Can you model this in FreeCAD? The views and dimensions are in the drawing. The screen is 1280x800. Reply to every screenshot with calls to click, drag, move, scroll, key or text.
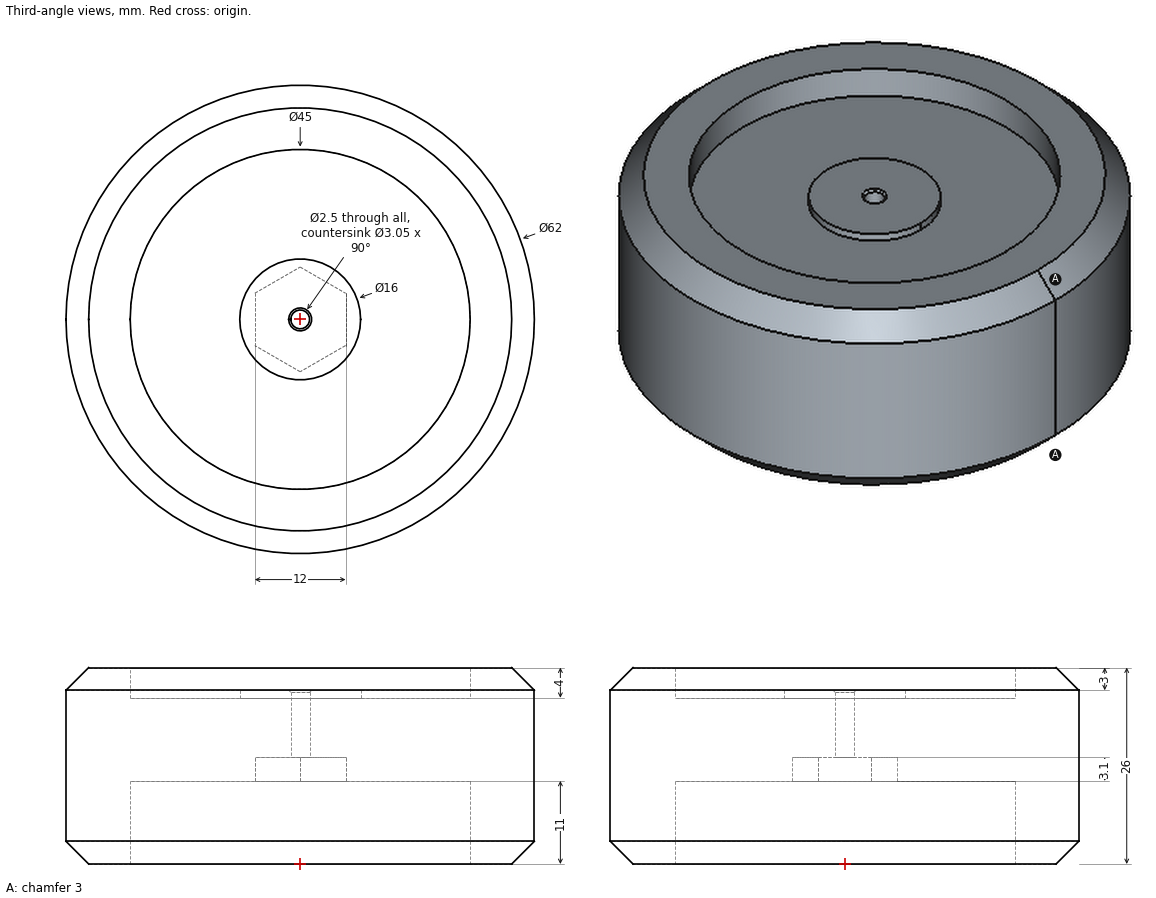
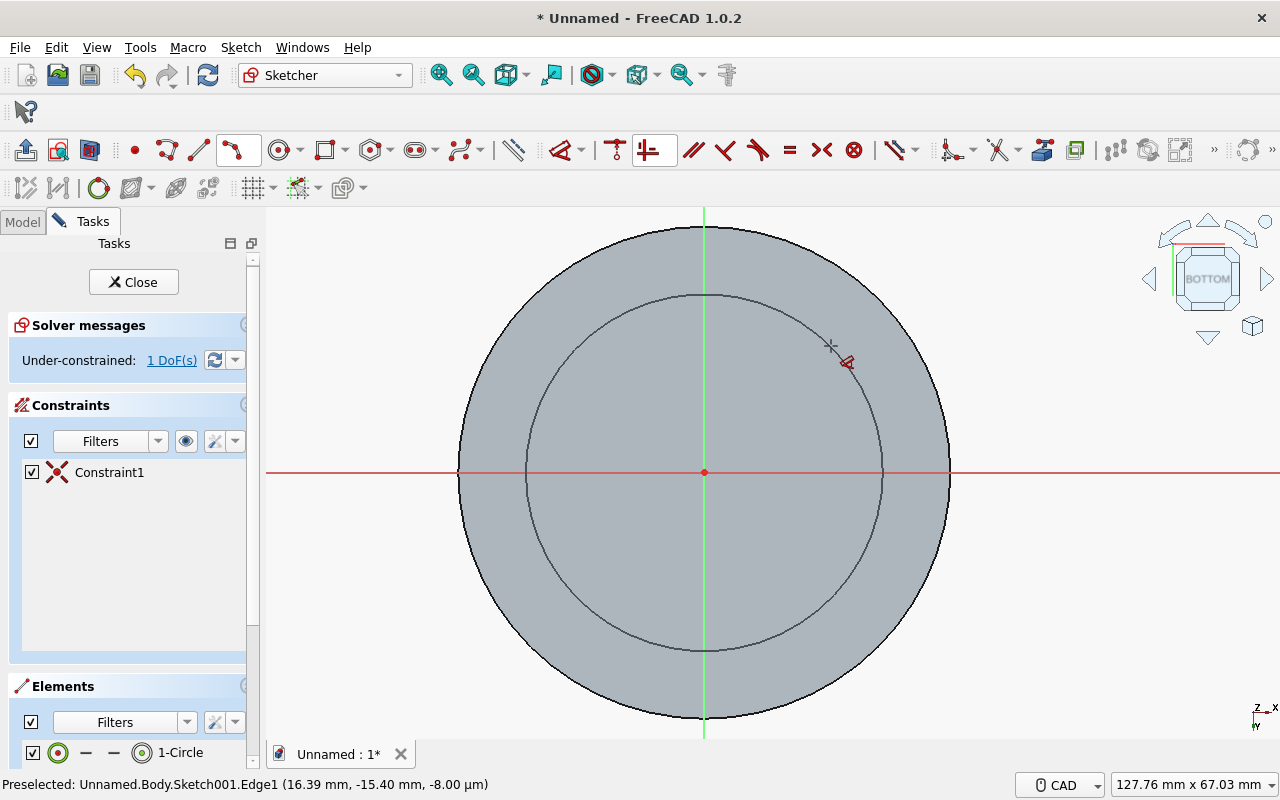
click(830, 346)
click(853, 323)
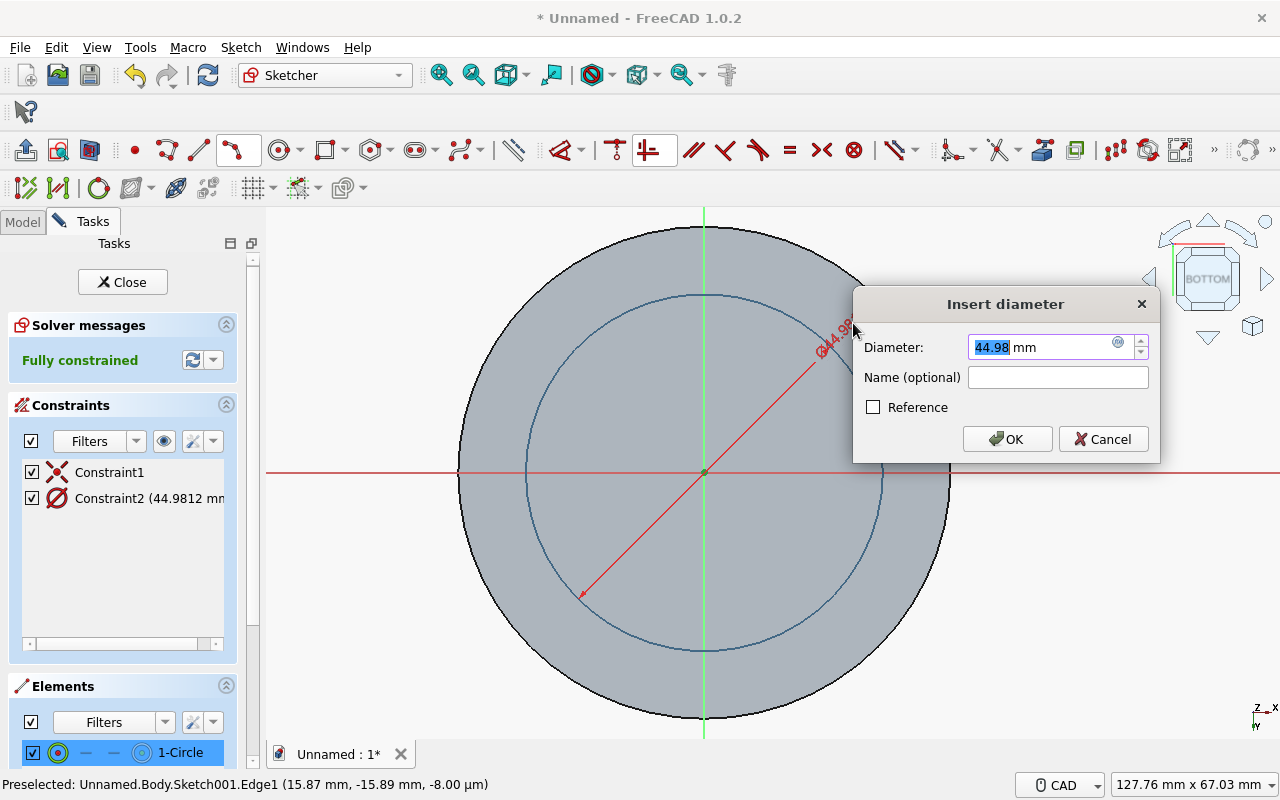
text(45)
key(Return)
key(Escape)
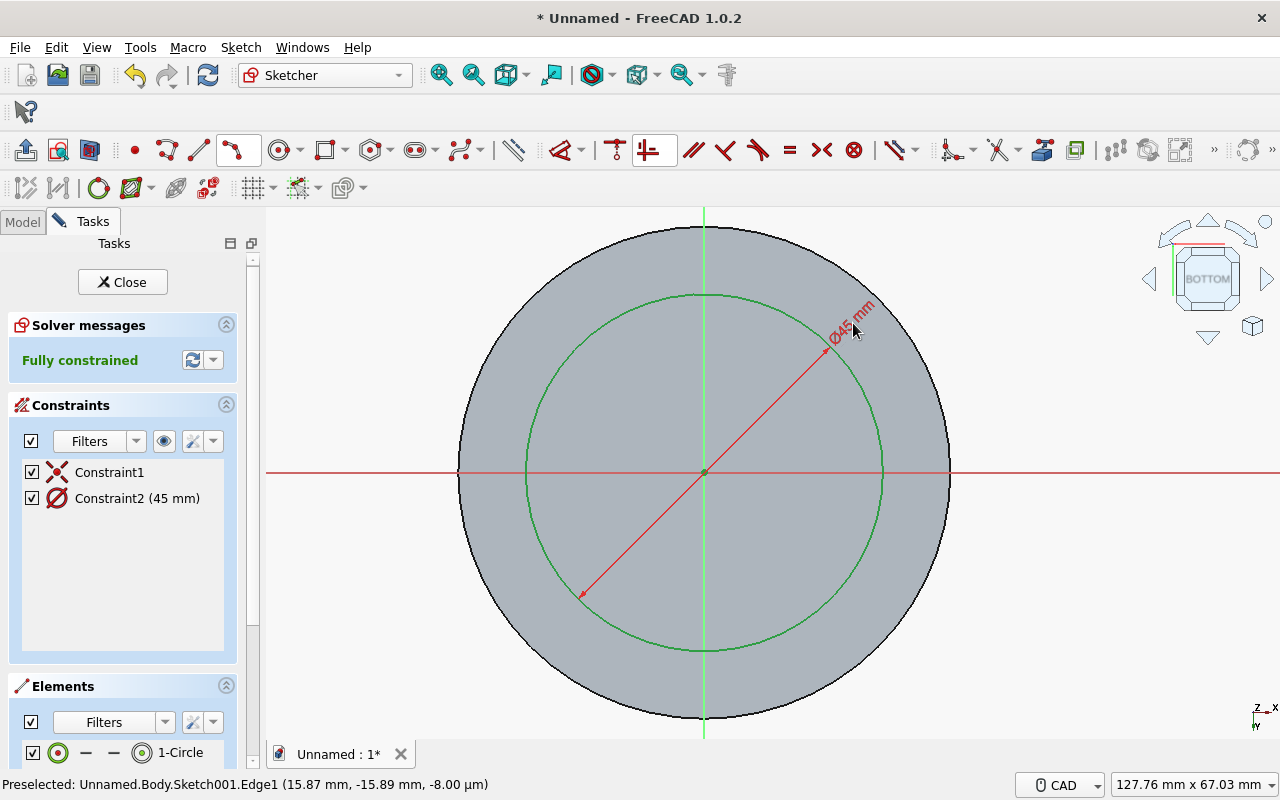
click(123, 282)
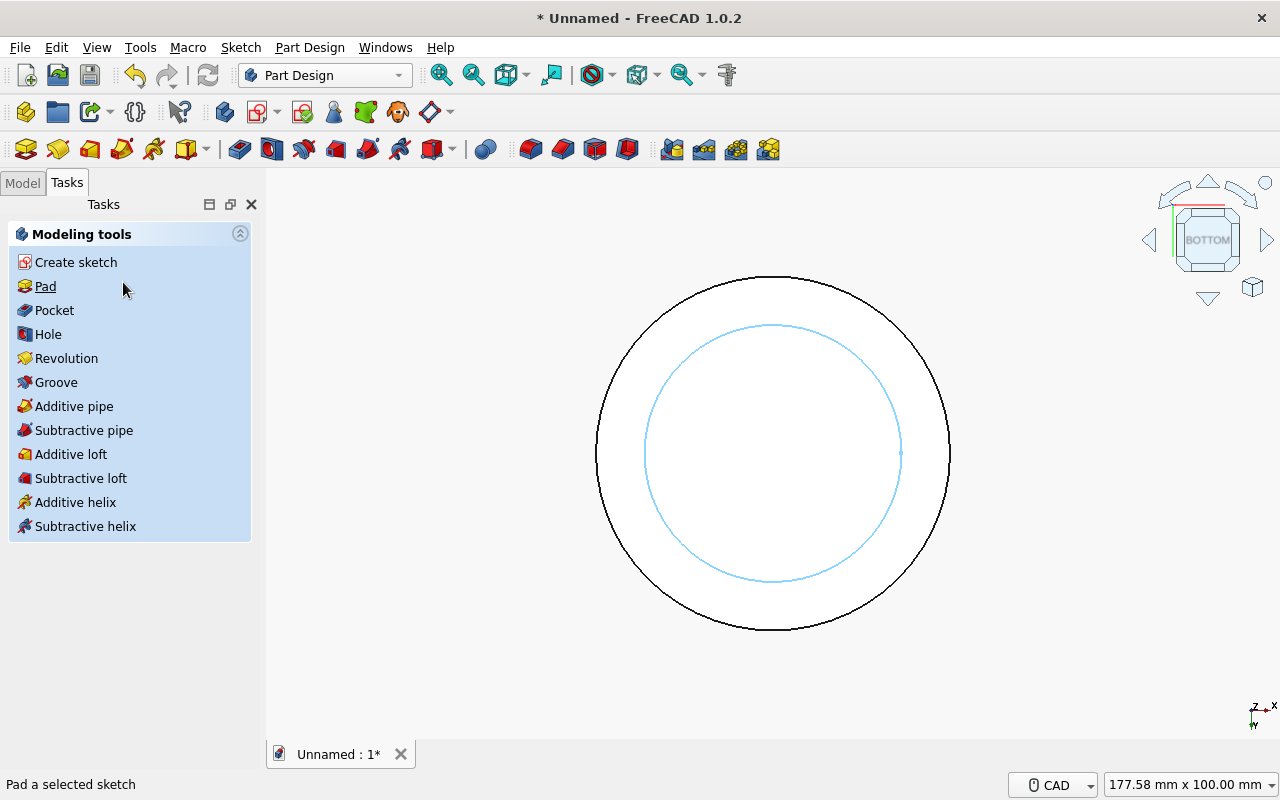
click(240, 150)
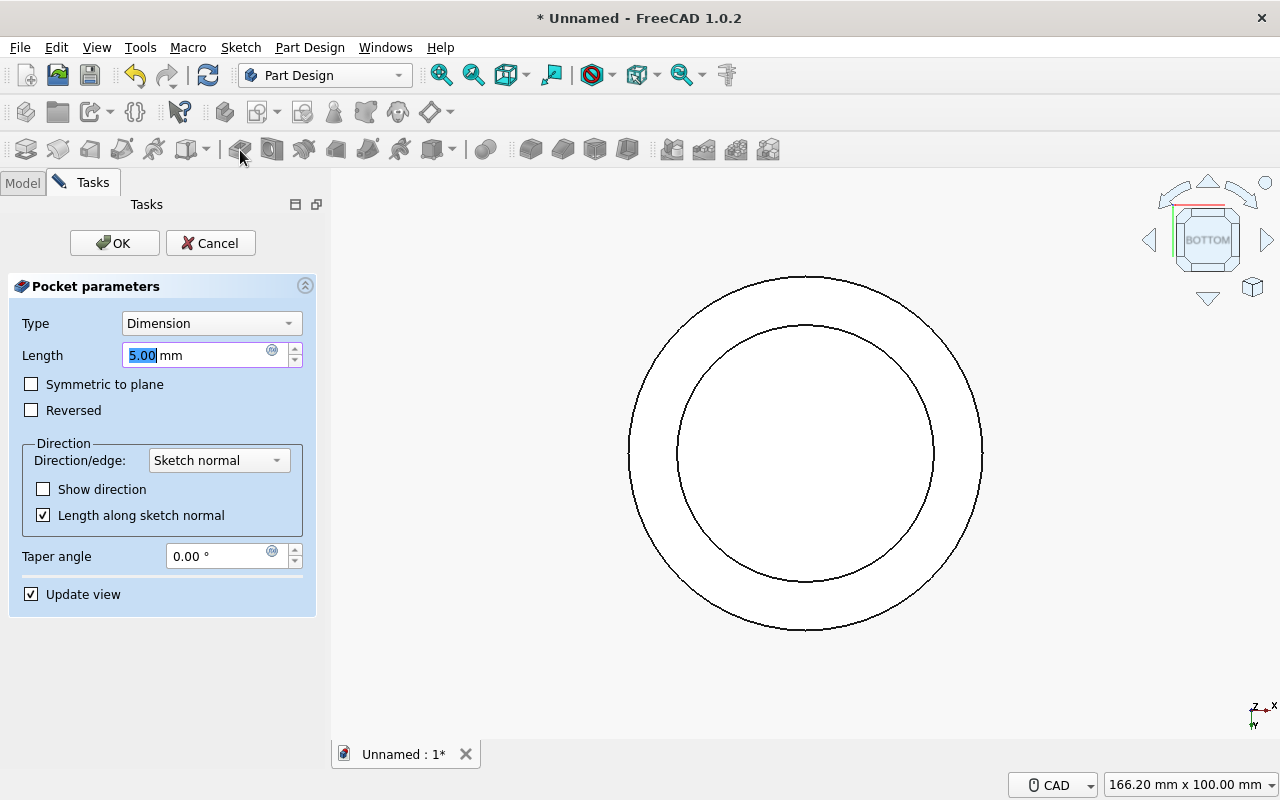
text(11)
key(Tab)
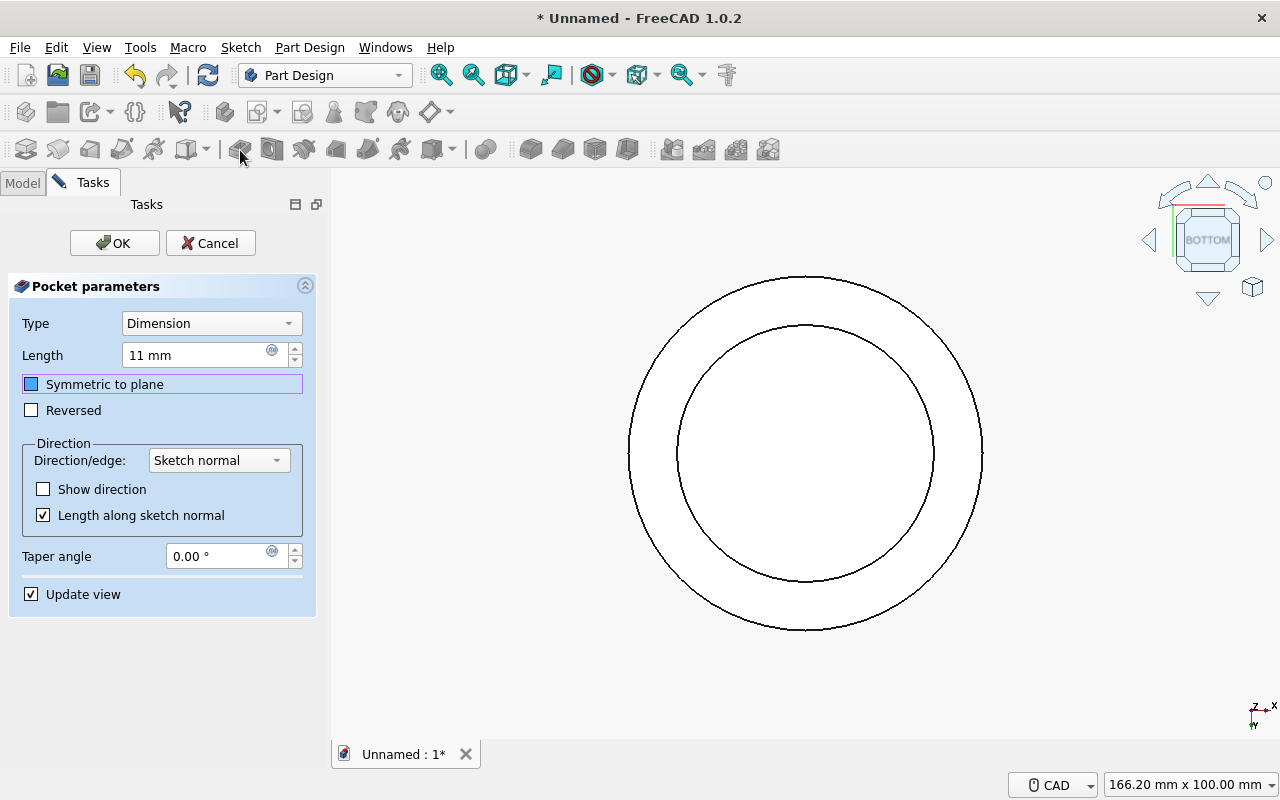
click(115, 243)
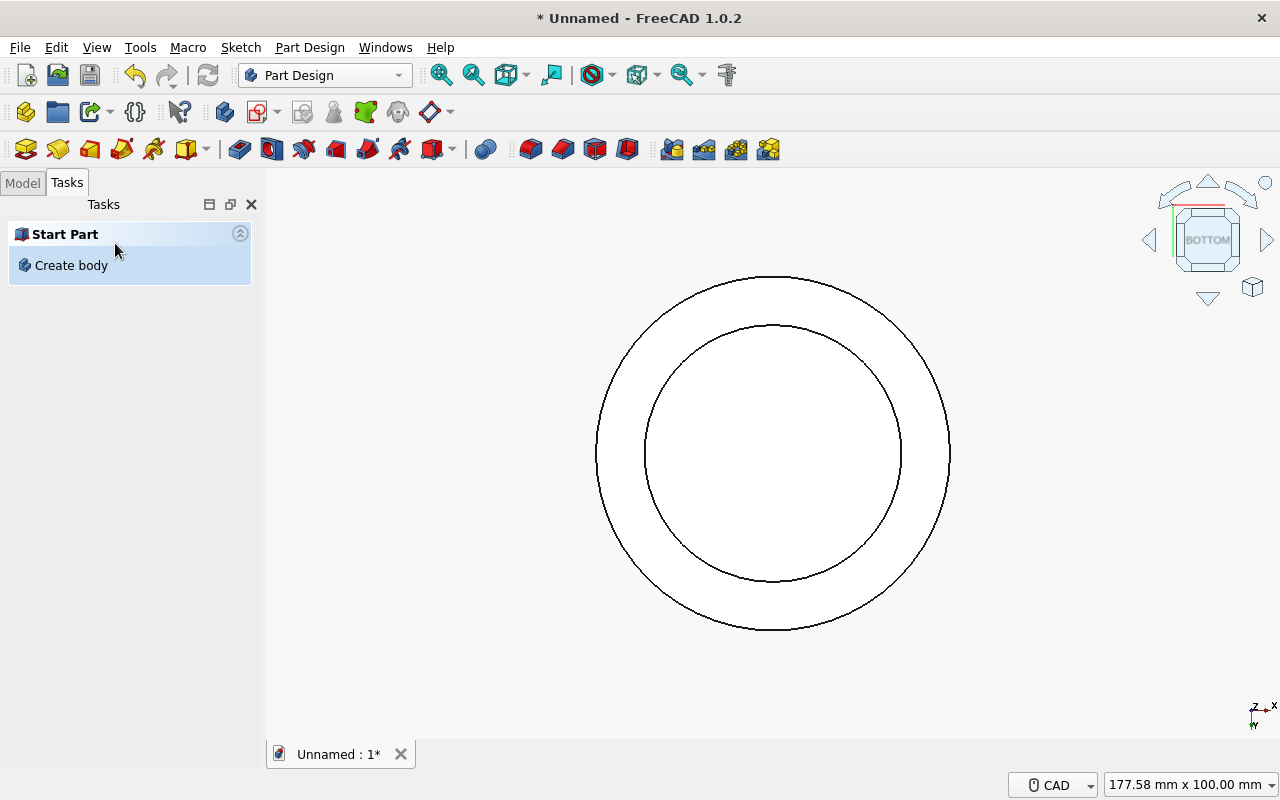
click(773, 453)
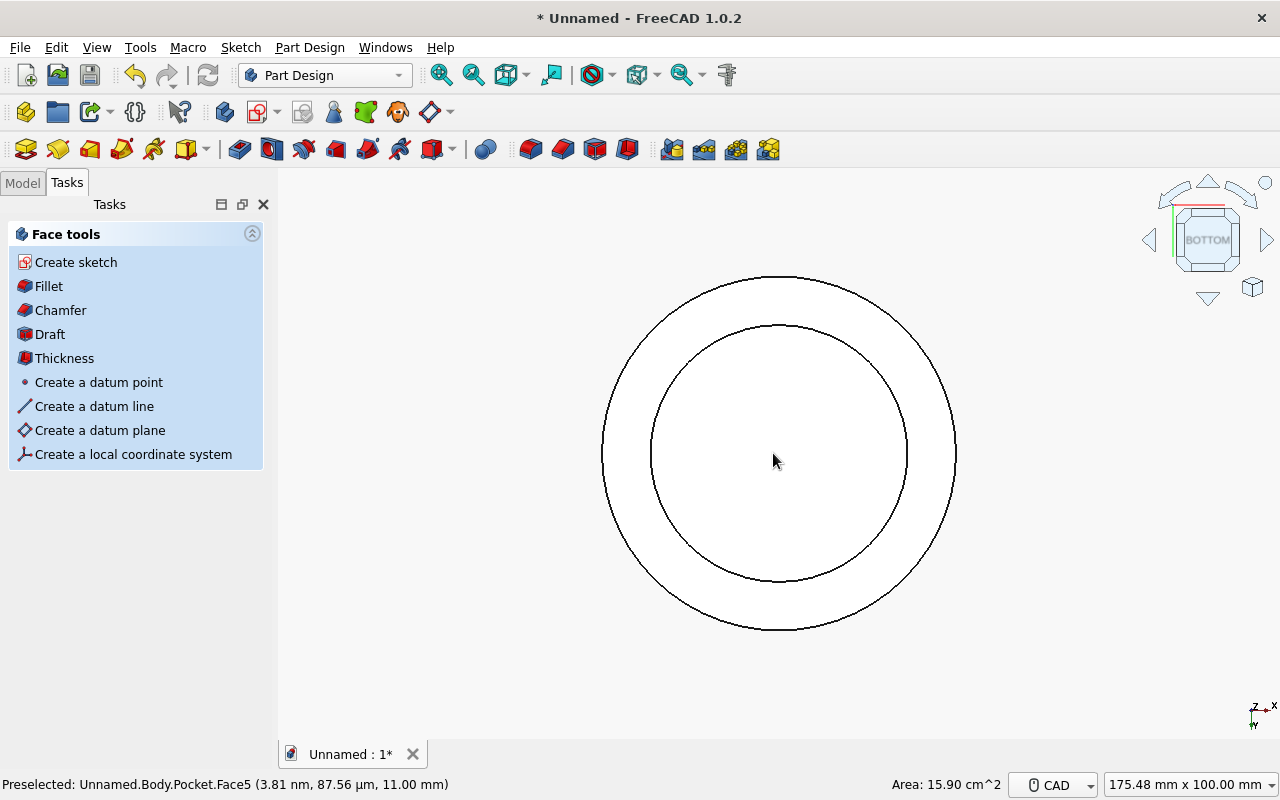
click(258, 112)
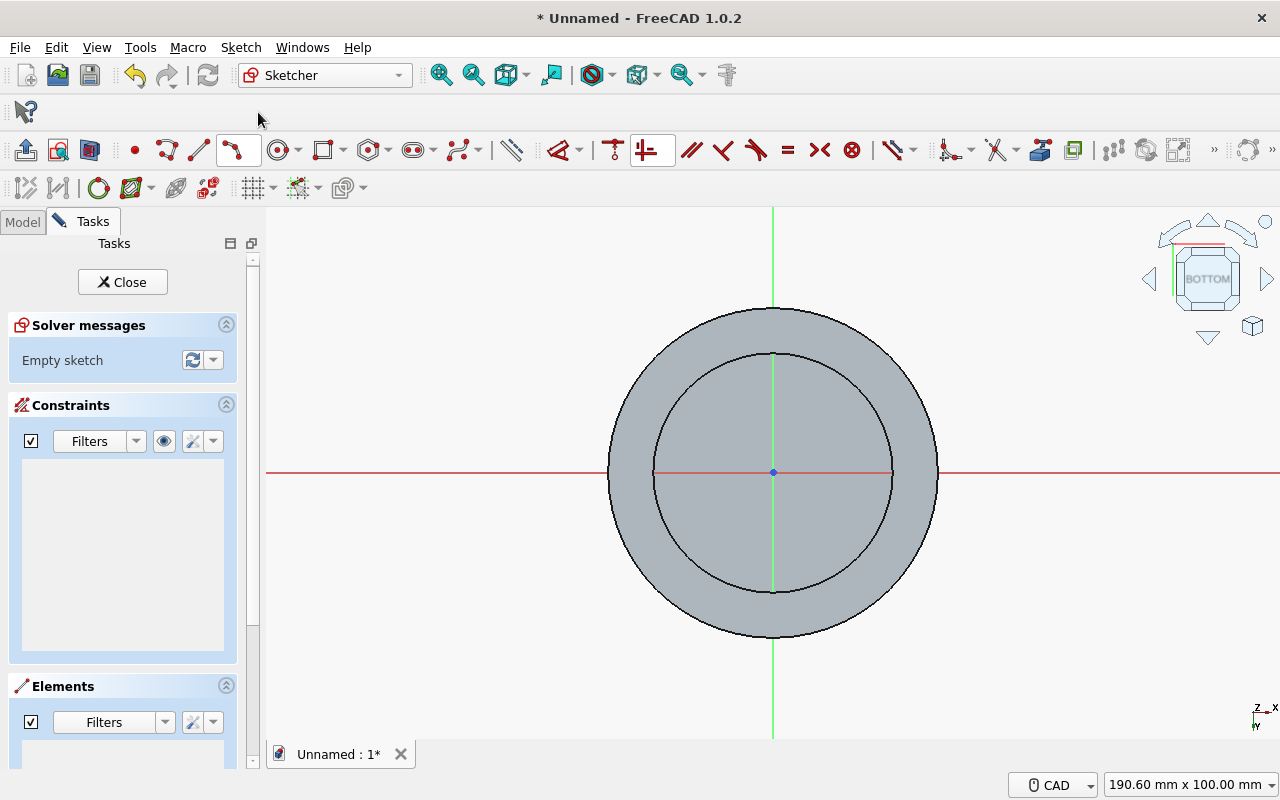
click(90, 150)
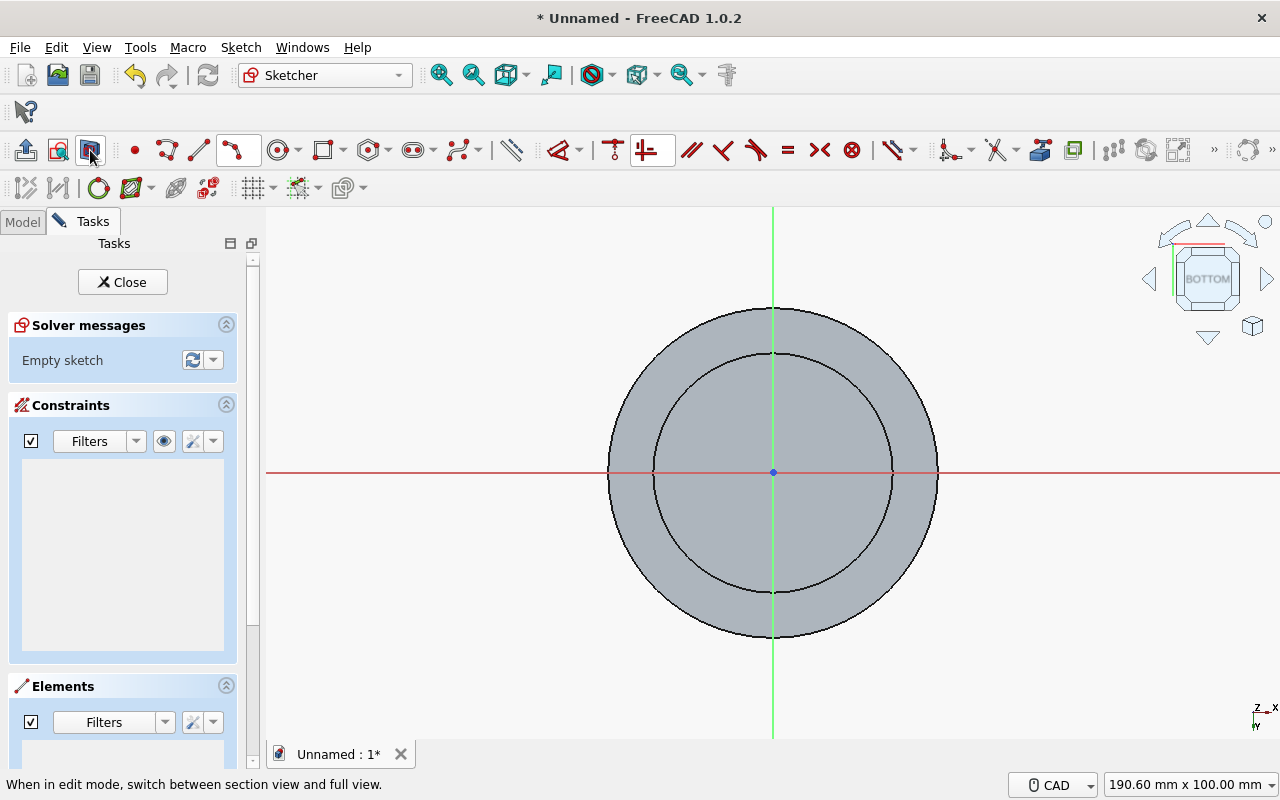
scroll(790, 473, up, 8)